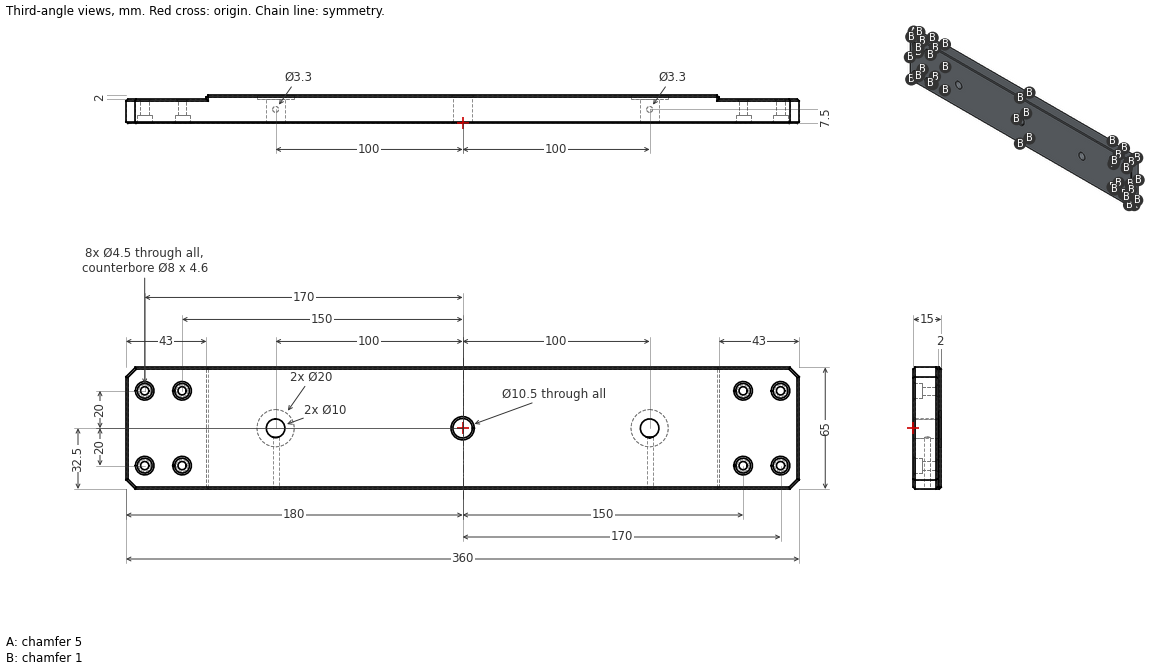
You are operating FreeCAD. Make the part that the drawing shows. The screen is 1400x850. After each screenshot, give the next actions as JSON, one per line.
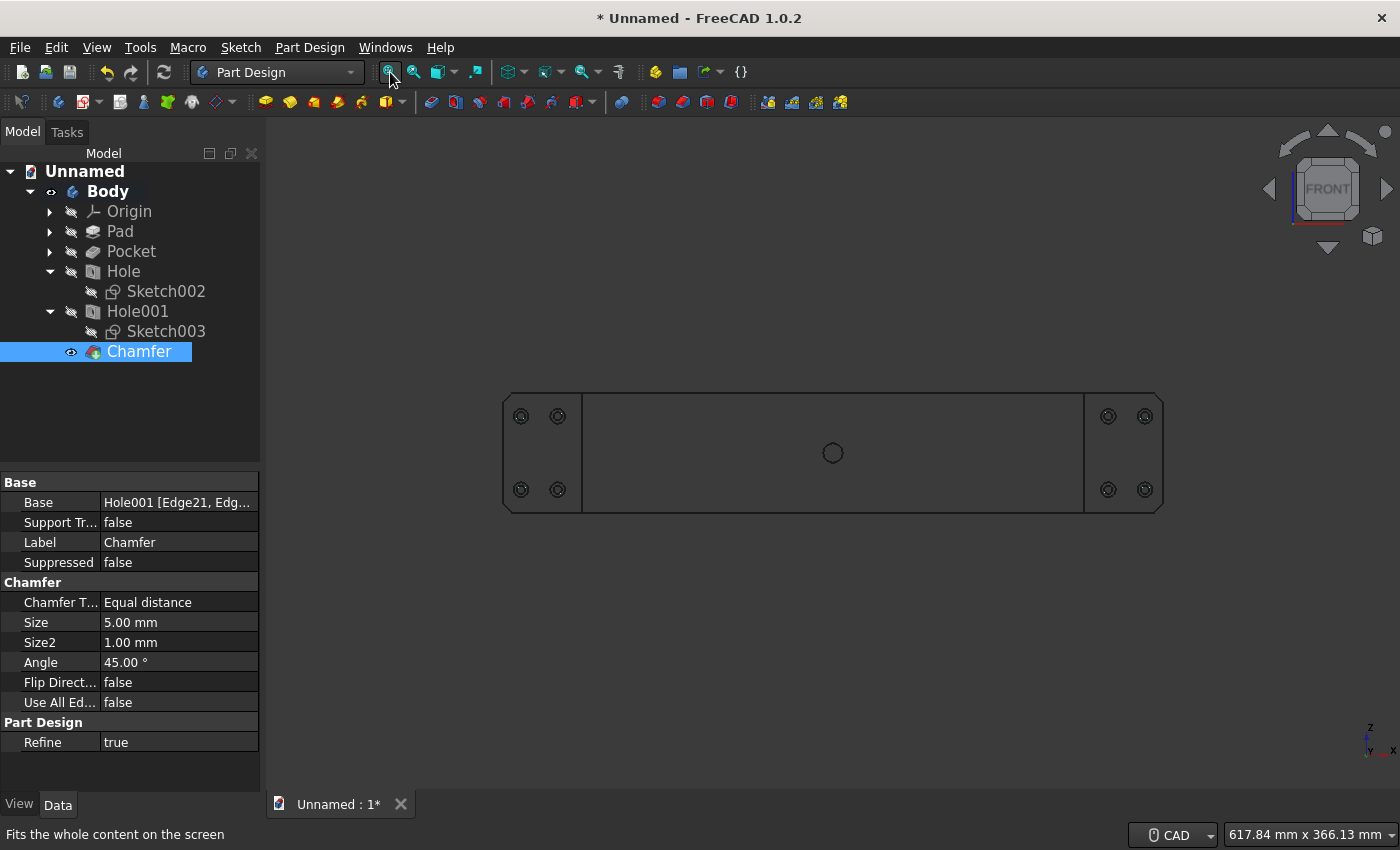
{"action": "key", "text": "3"}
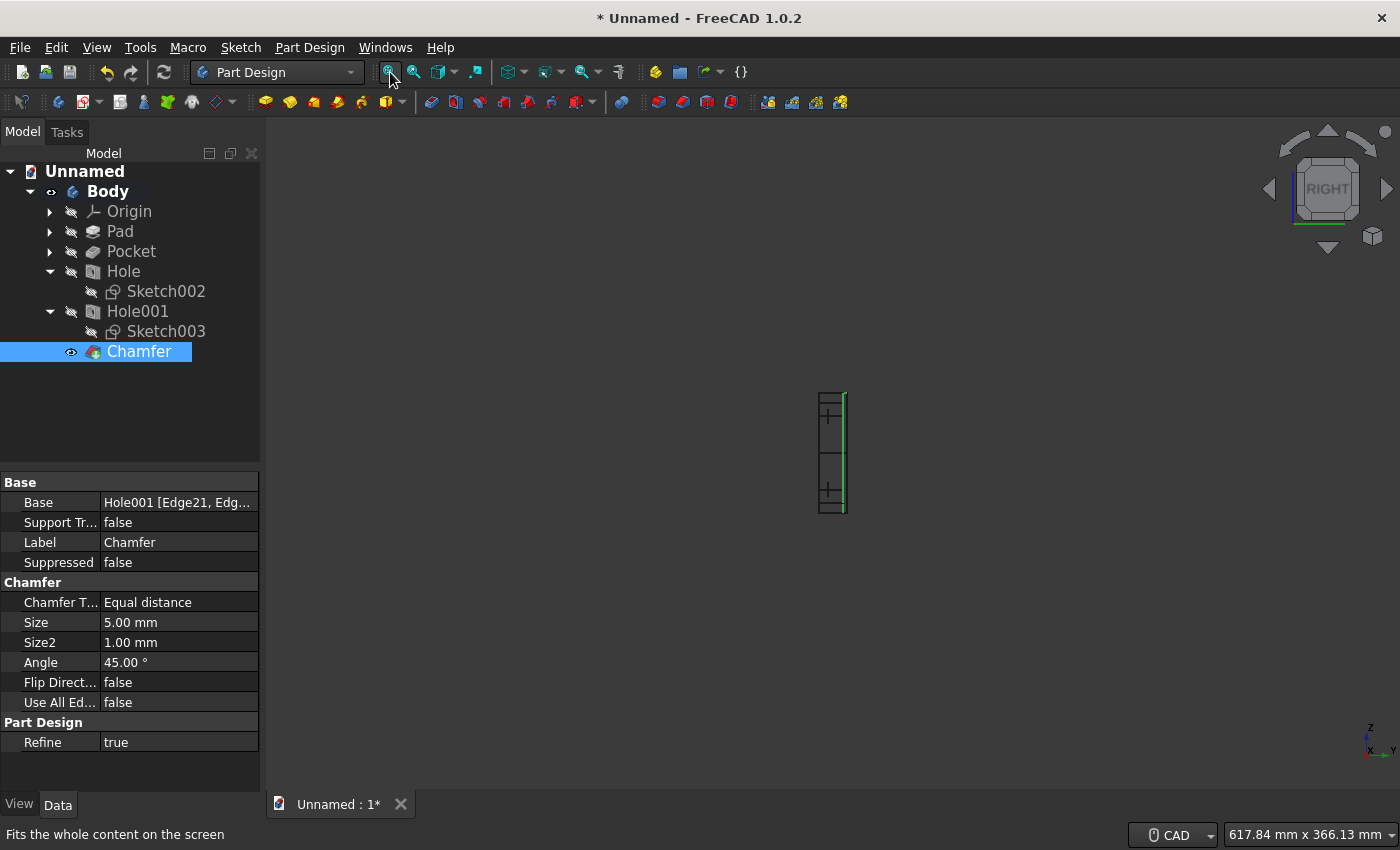
{"action": "left_click", "coordinate": [390, 72]}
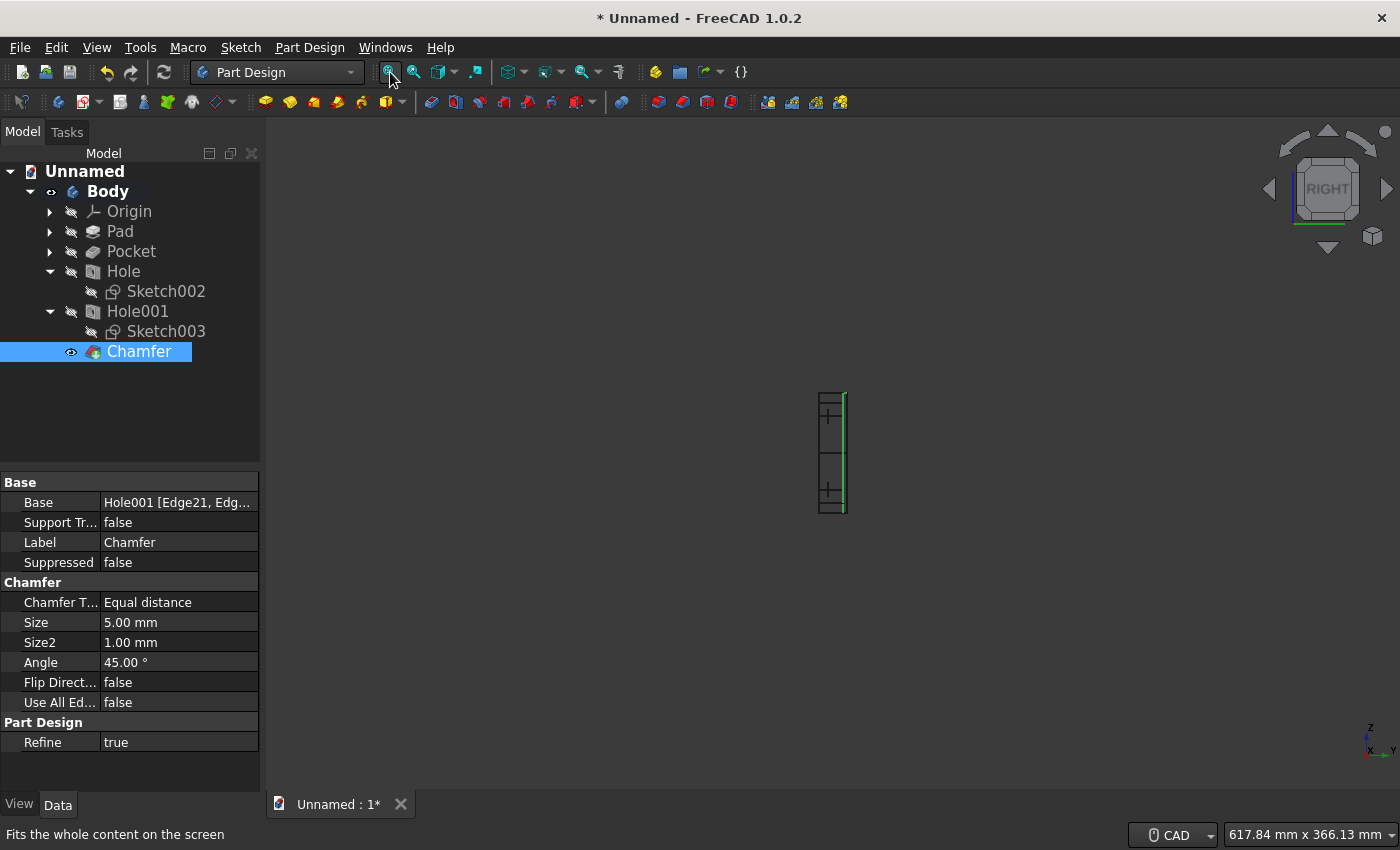
{"action": "scroll", "coordinate": [845, 512], "scroll_direction": "up", "scroll_amount": 12}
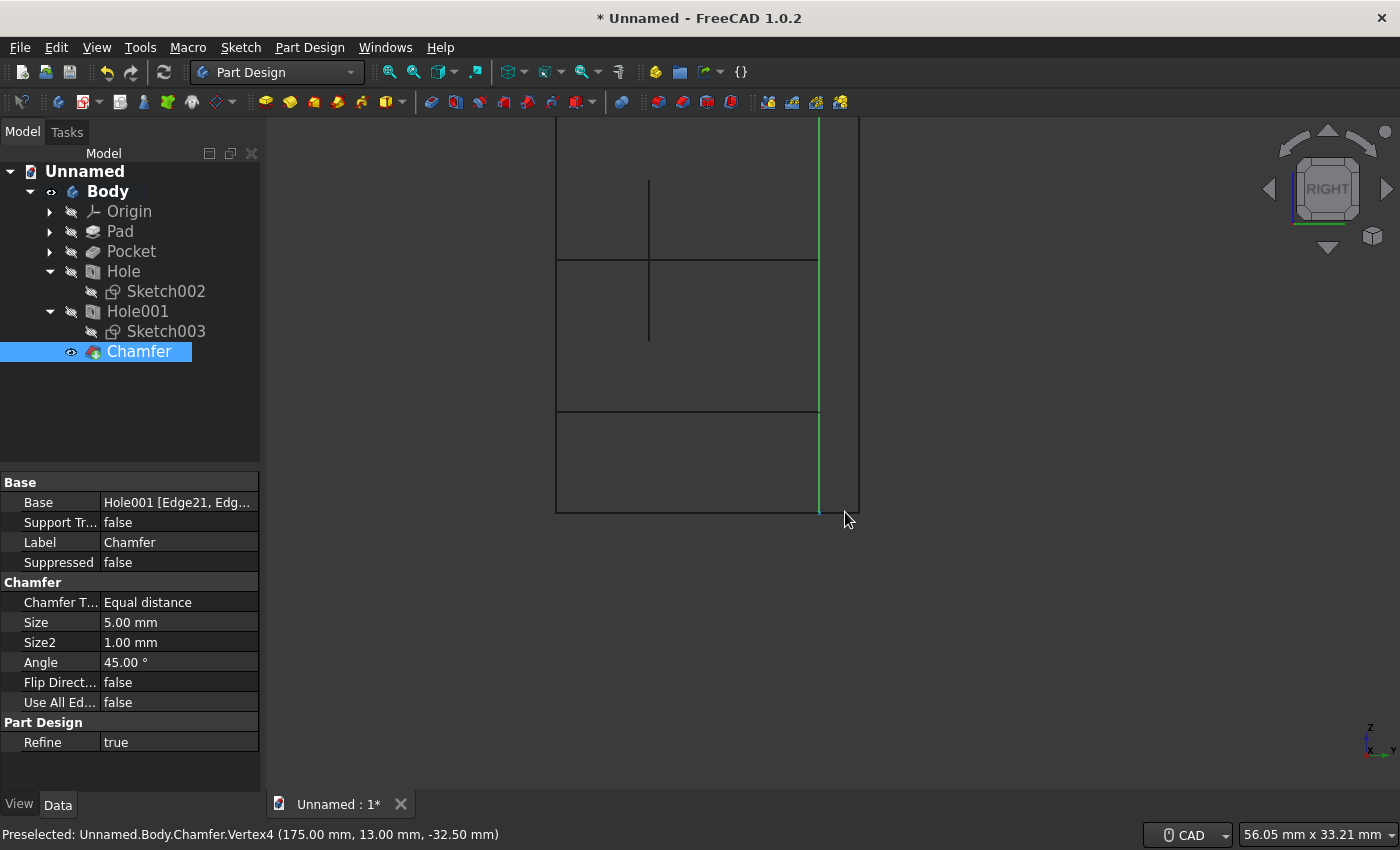
{"action": "left_click", "coordinate": [839, 512], "text": "ctrl"}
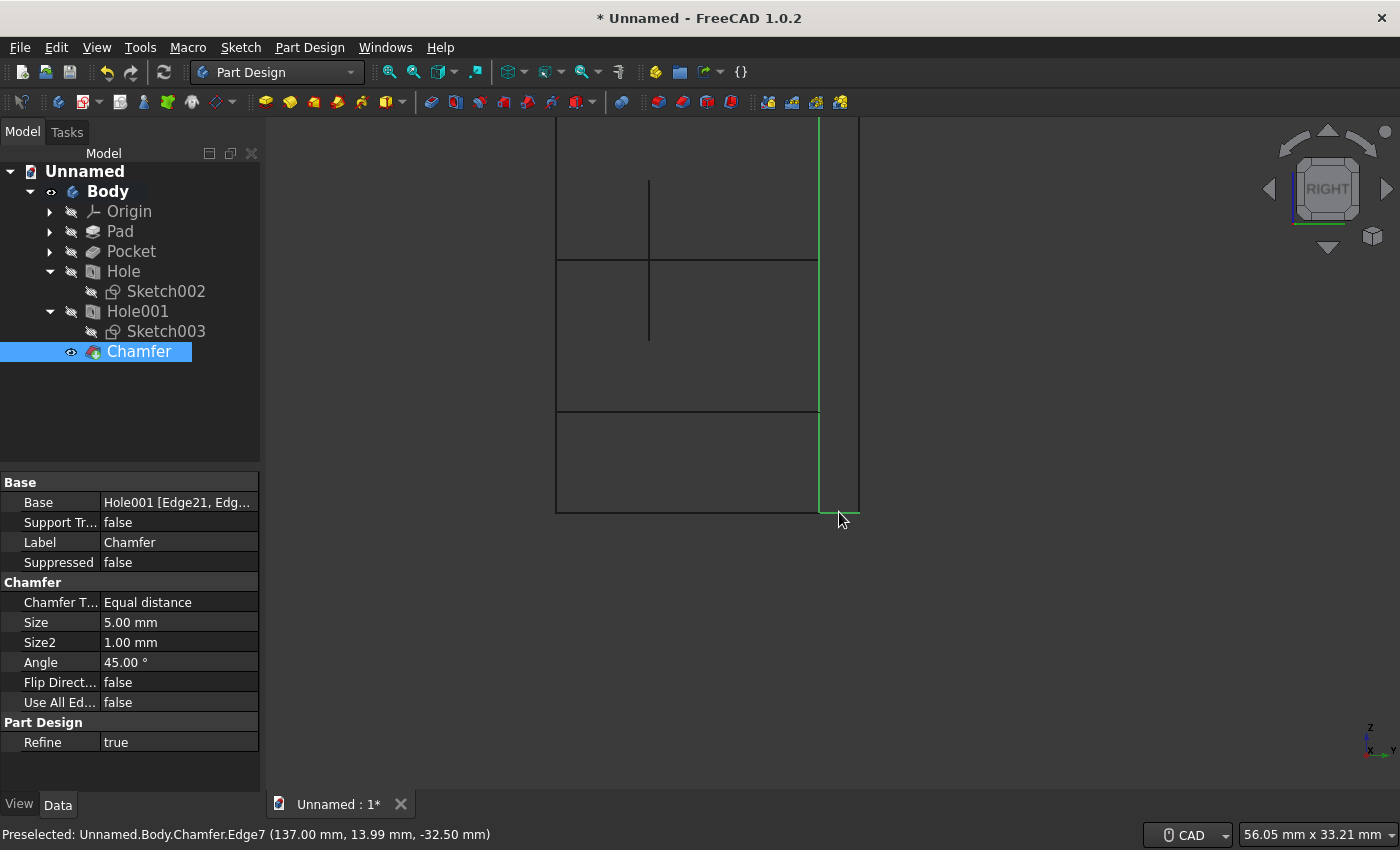
{"action": "key", "text": "v 1"}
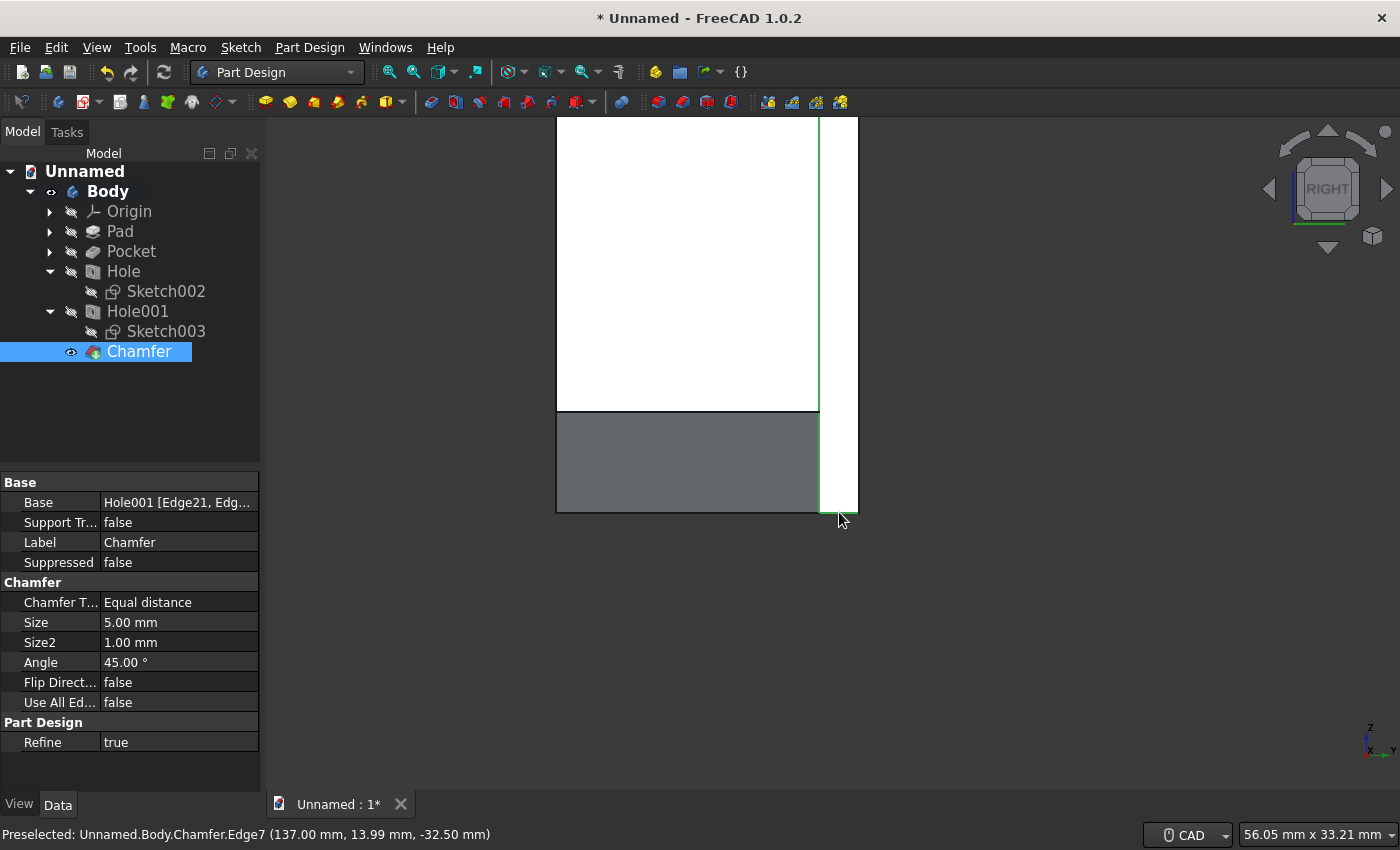
{"action": "left_click", "coordinate": [684, 102]}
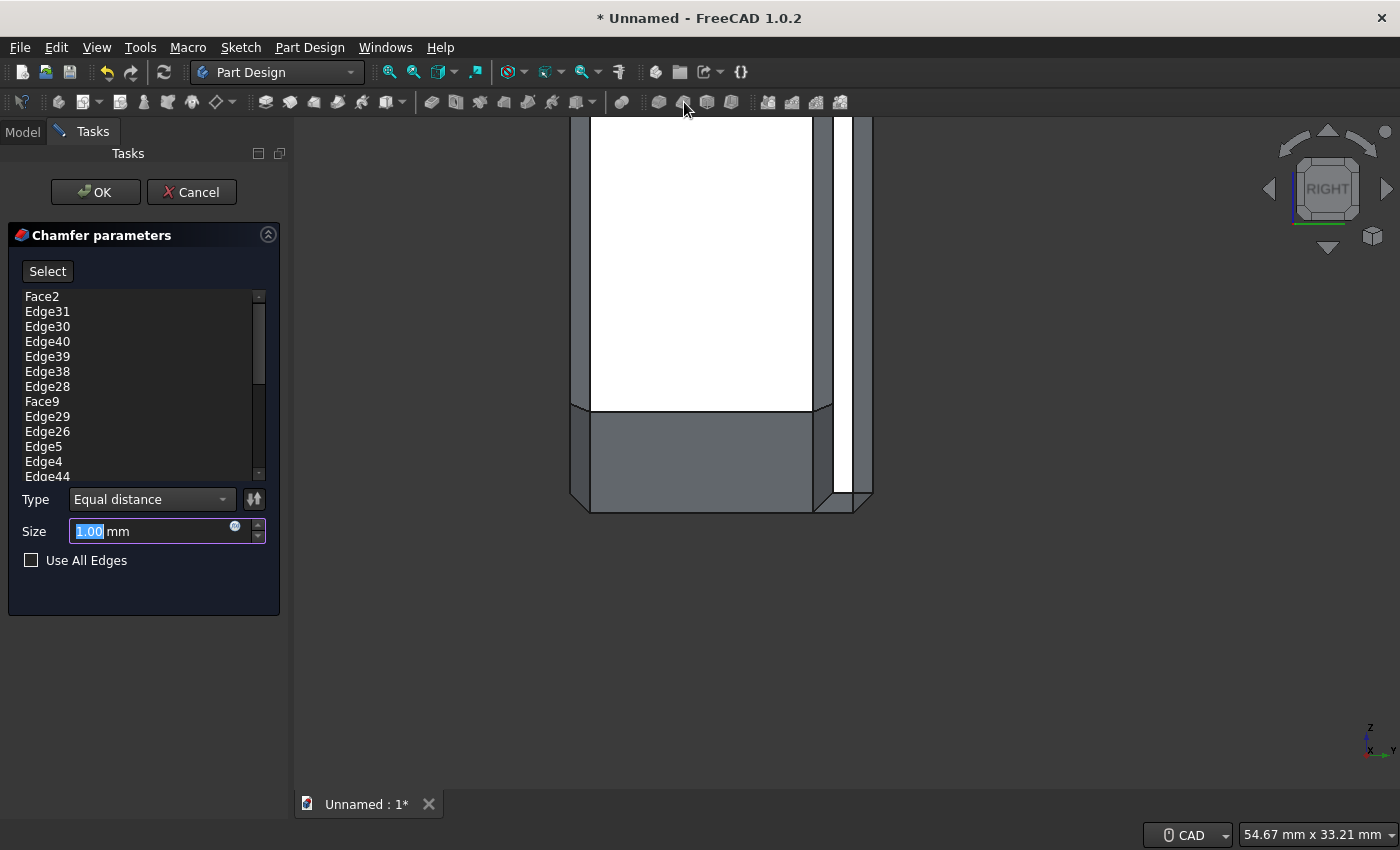
{"action": "type", "text": "1"}
{"action": "key", "text": "Tab"}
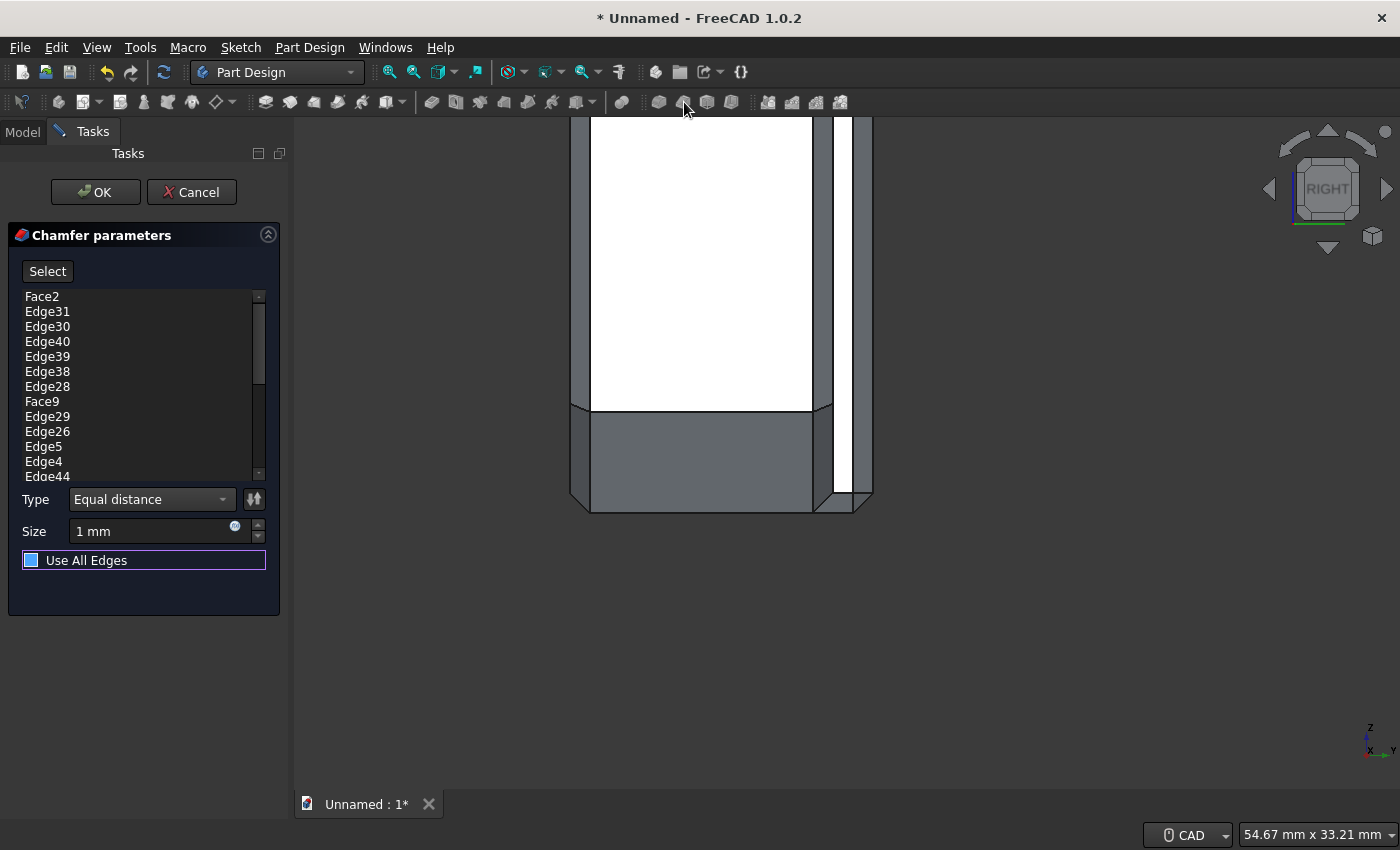
{"action": "left_click", "coordinate": [96, 192]}